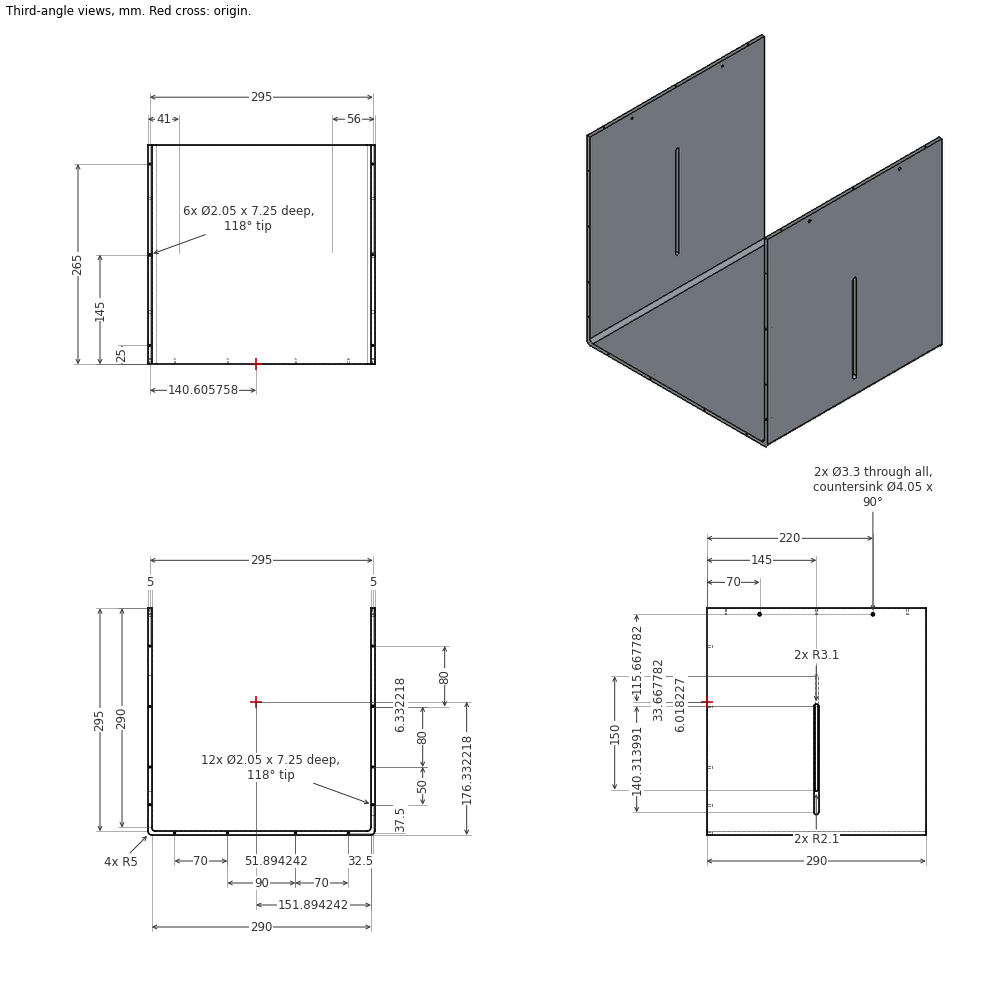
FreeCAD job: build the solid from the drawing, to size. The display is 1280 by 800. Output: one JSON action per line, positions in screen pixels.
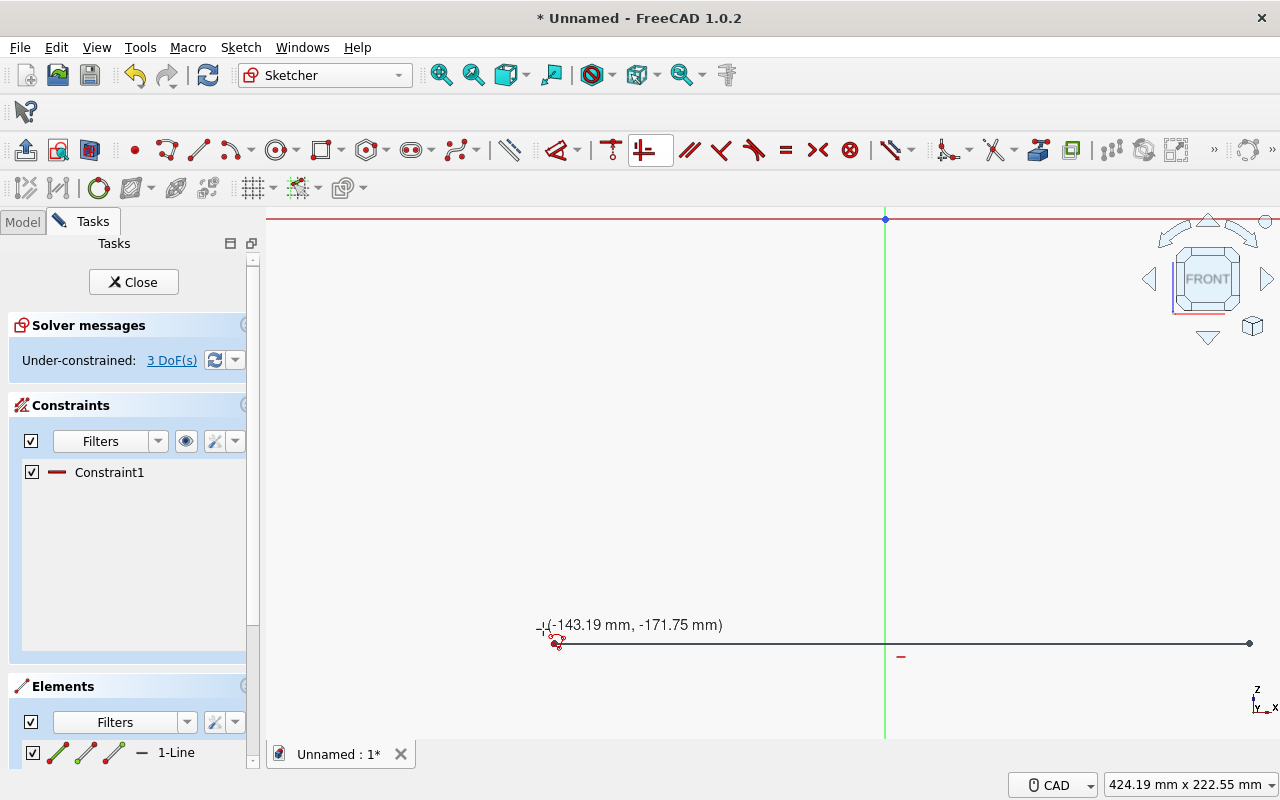
{"action": "scroll", "coordinate": [544, 629], "scroll_direction": "down", "scroll_amount": 4}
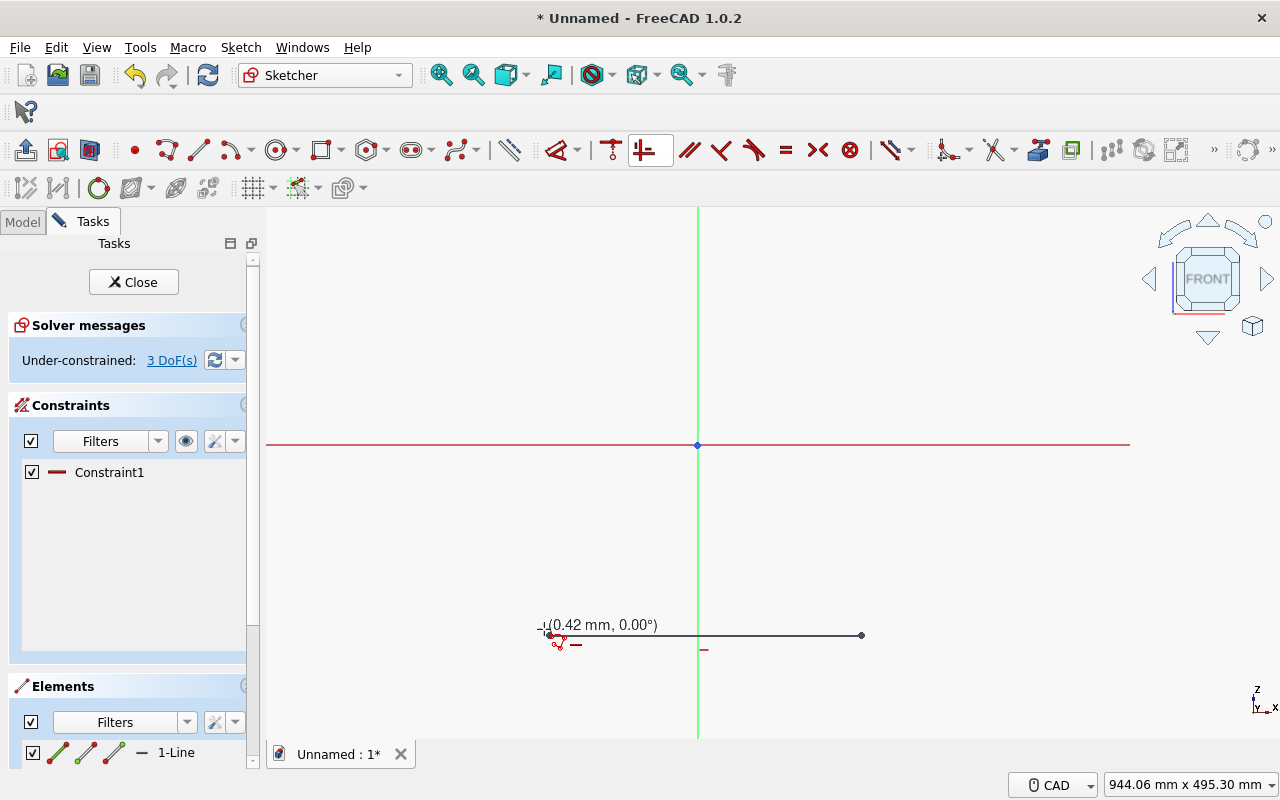
{"action": "left_click", "coordinate": [544, 313]}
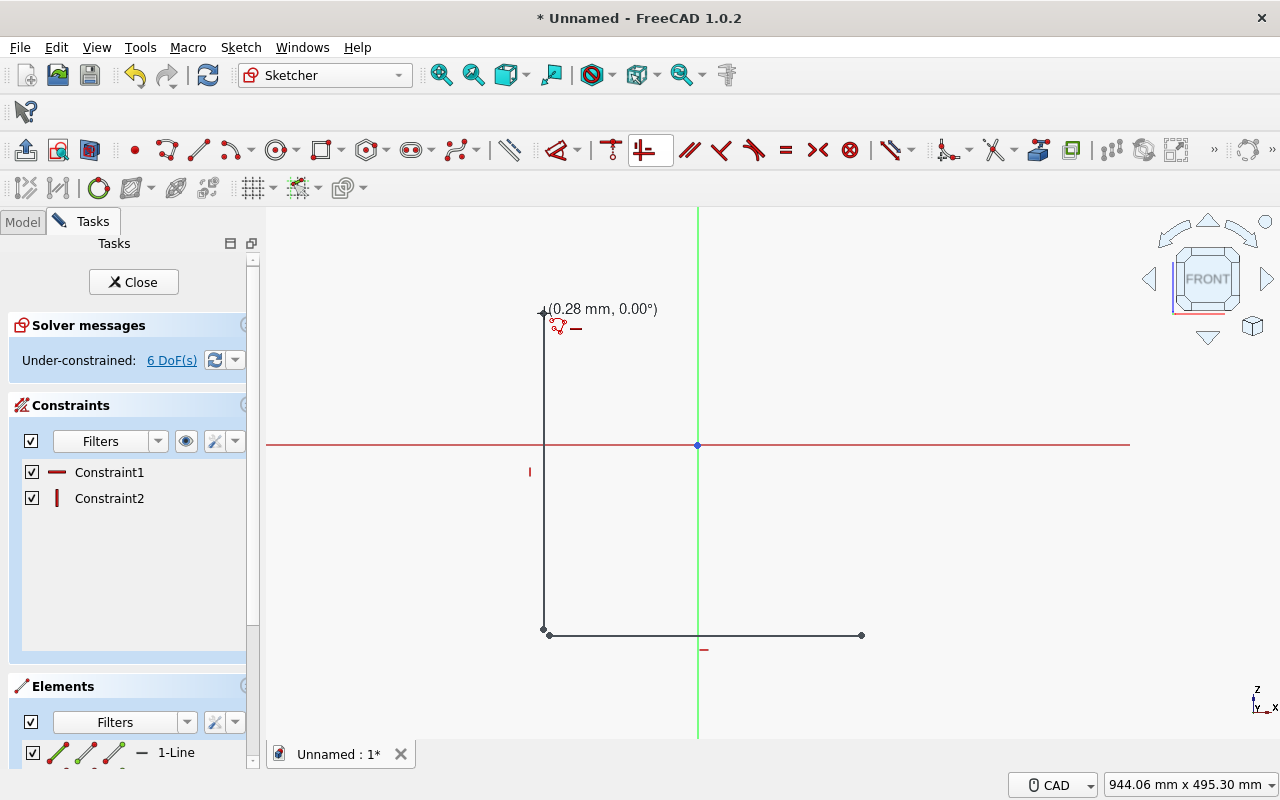
{"action": "scroll", "coordinate": [549, 313], "scroll_direction": "up", "scroll_amount": 6}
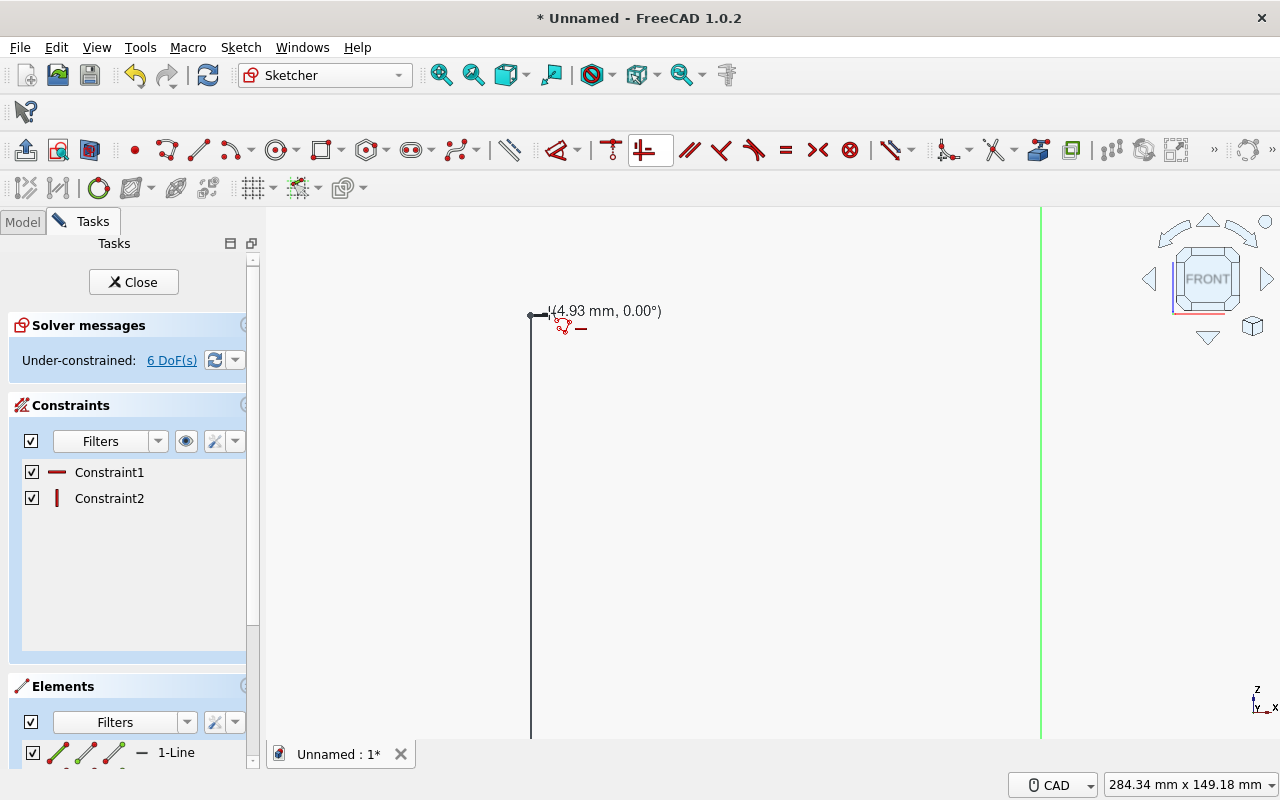
{"action": "left_click", "coordinate": [549, 313]}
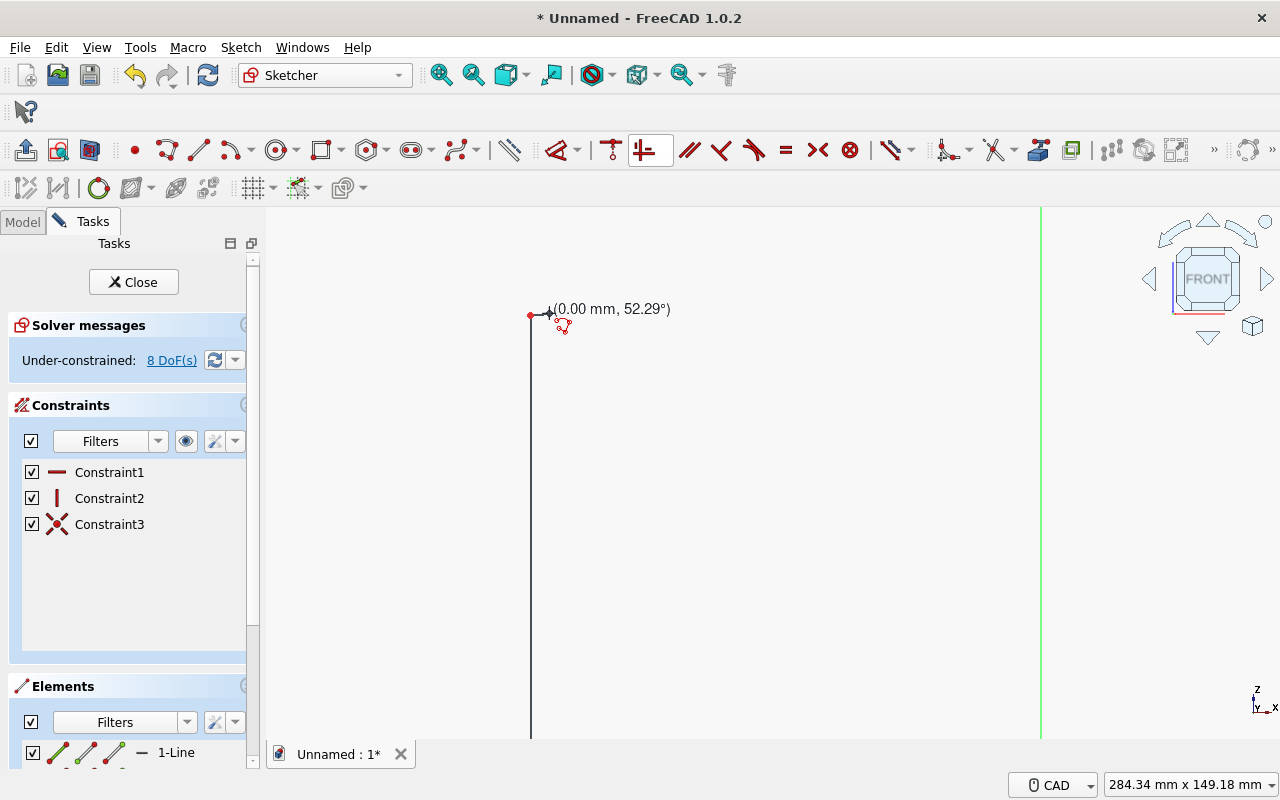
{"action": "scroll", "coordinate": [549, 312], "scroll_direction": "down", "scroll_amount": 6}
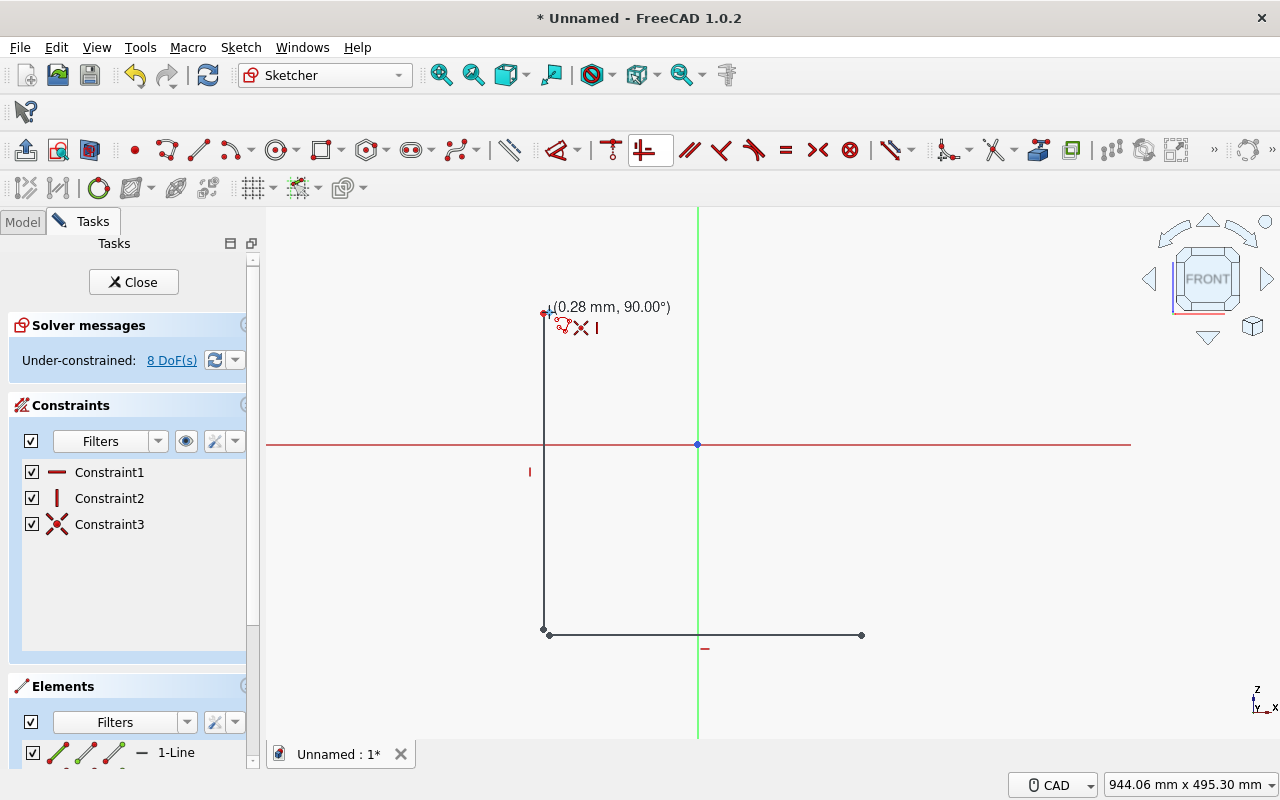
{"action": "scroll", "coordinate": [549, 623], "scroll_direction": "up", "scroll_amount": 6}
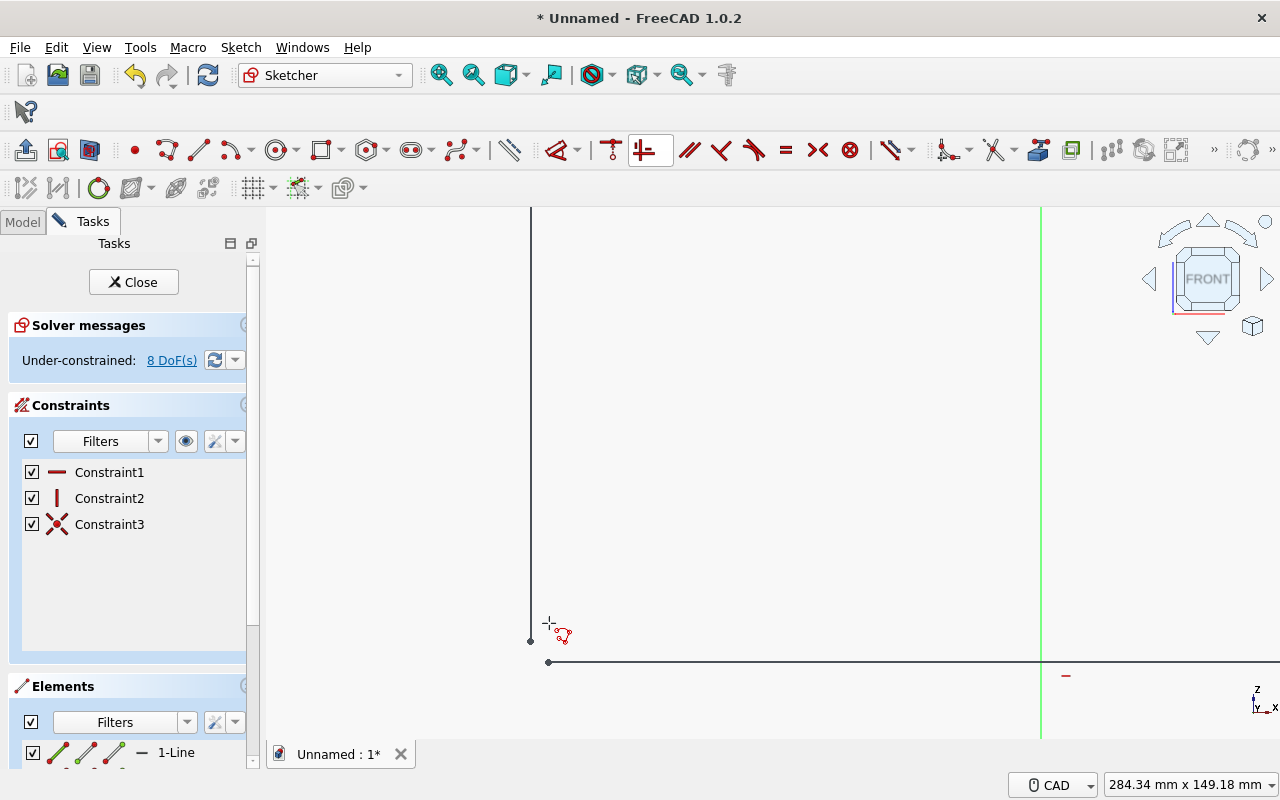
{"action": "left_click", "coordinate": [549, 622]}
{"action": "right_click", "coordinate": [549, 622]}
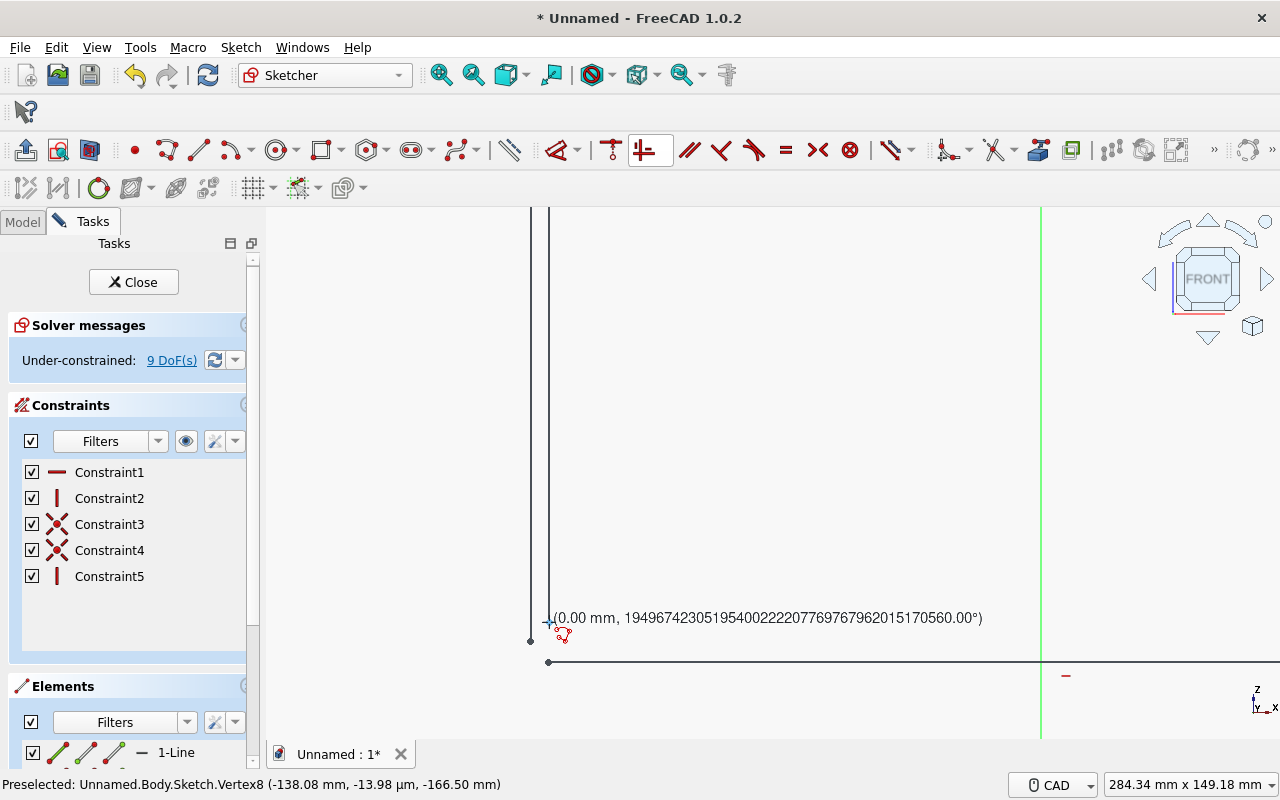
{"action": "left_click", "coordinate": [200, 150]}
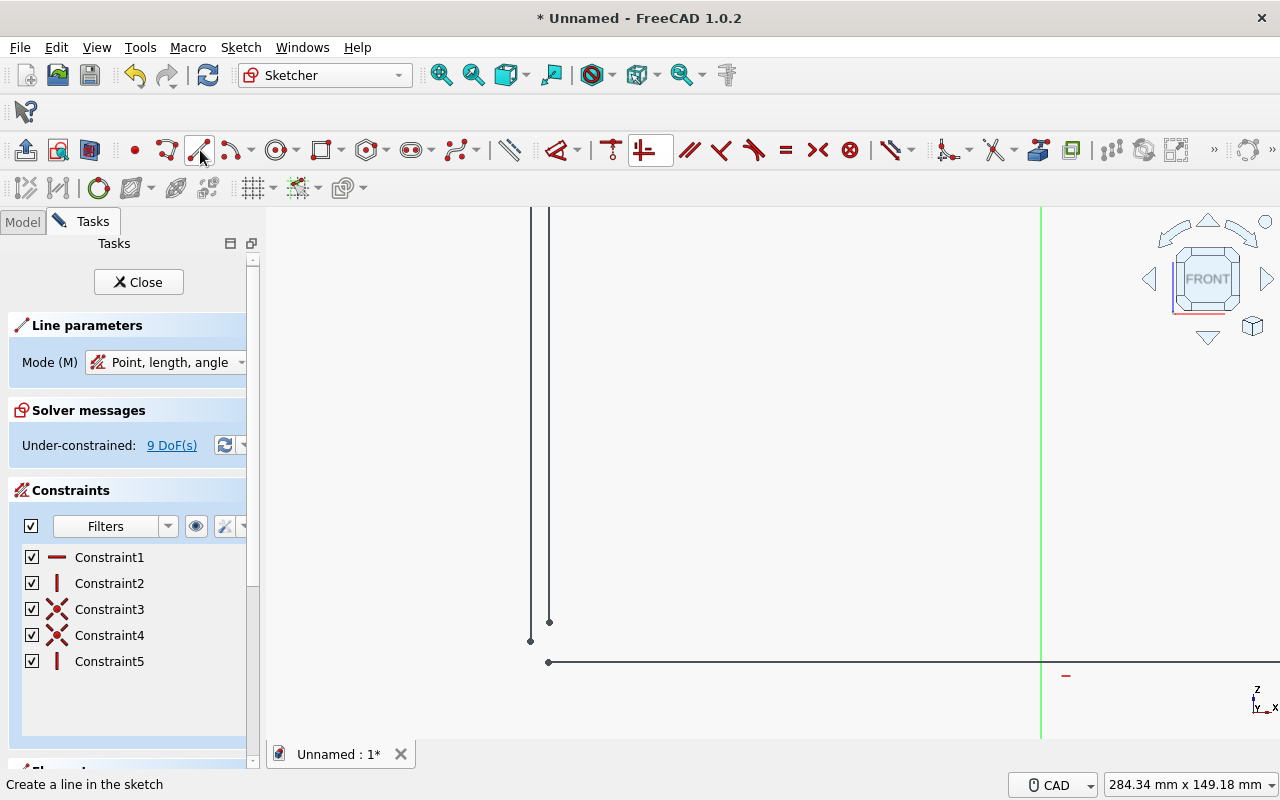
{"action": "left_click", "coordinate": [567, 640]}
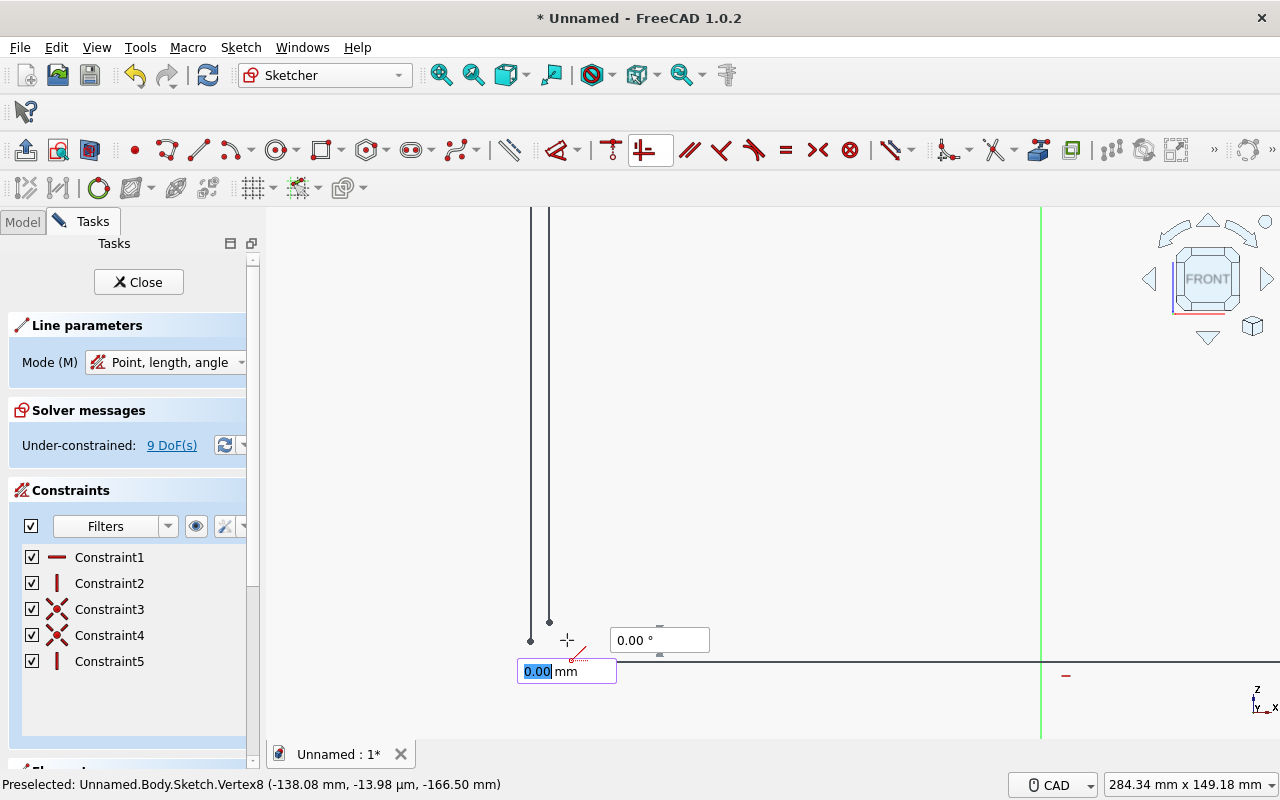
{"action": "scroll", "coordinate": [549, 624], "scroll_direction": "down", "scroll_amount": 6}